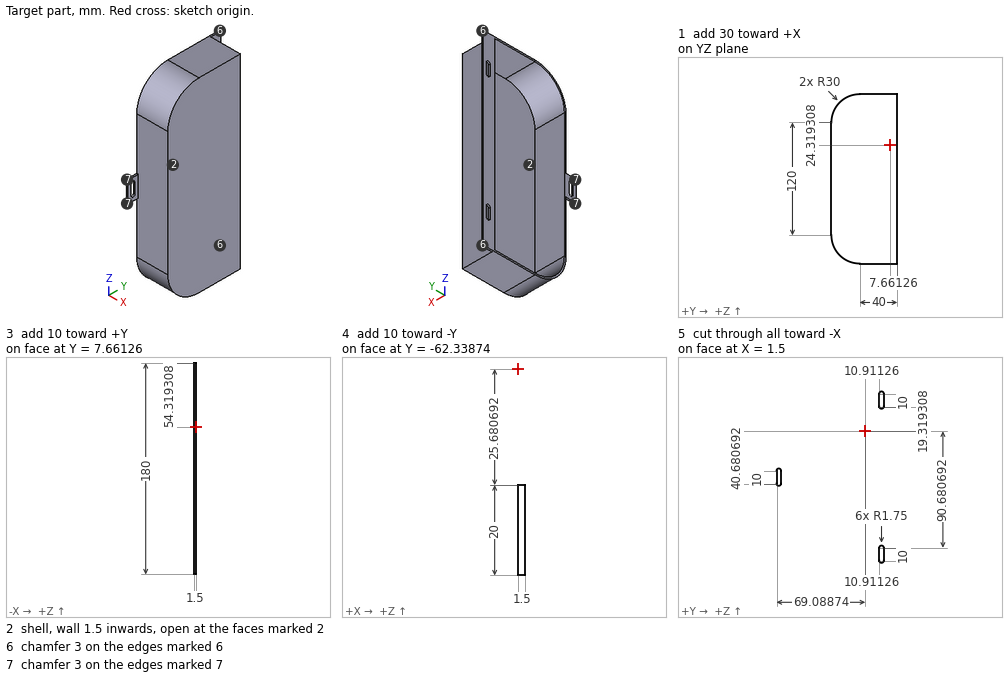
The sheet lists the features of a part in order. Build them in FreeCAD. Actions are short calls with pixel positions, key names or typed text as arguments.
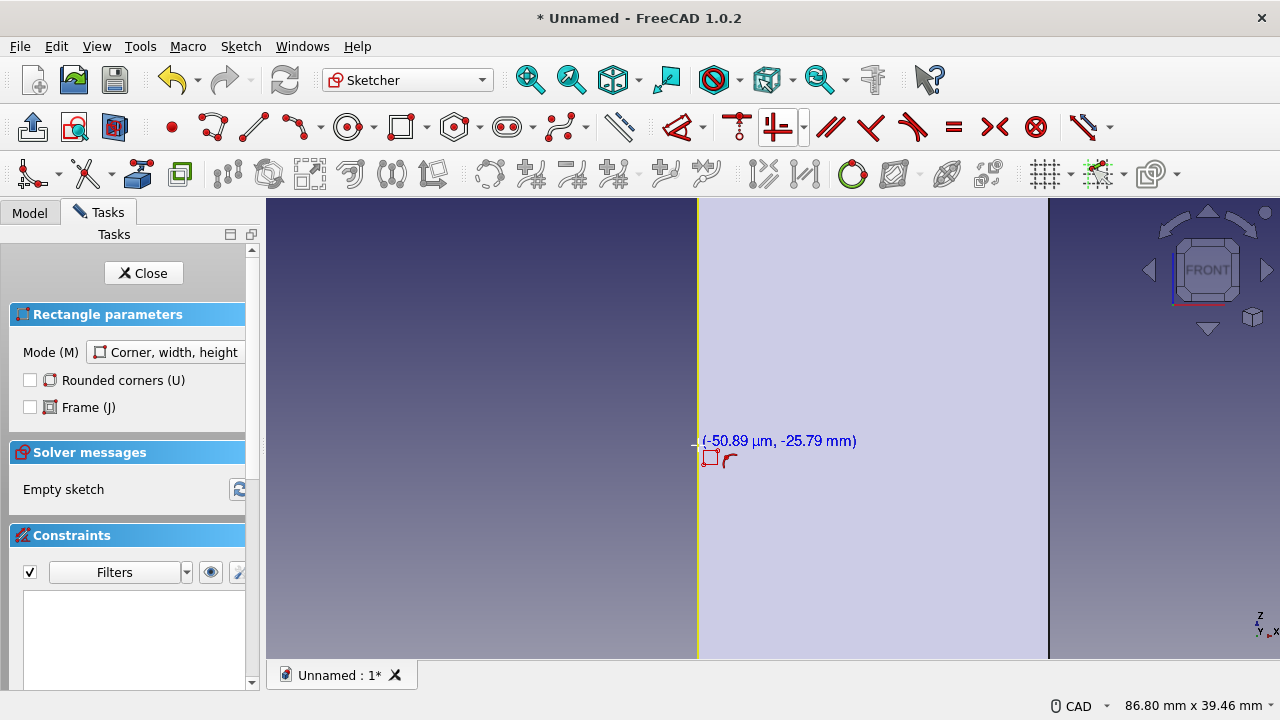
click(698, 445)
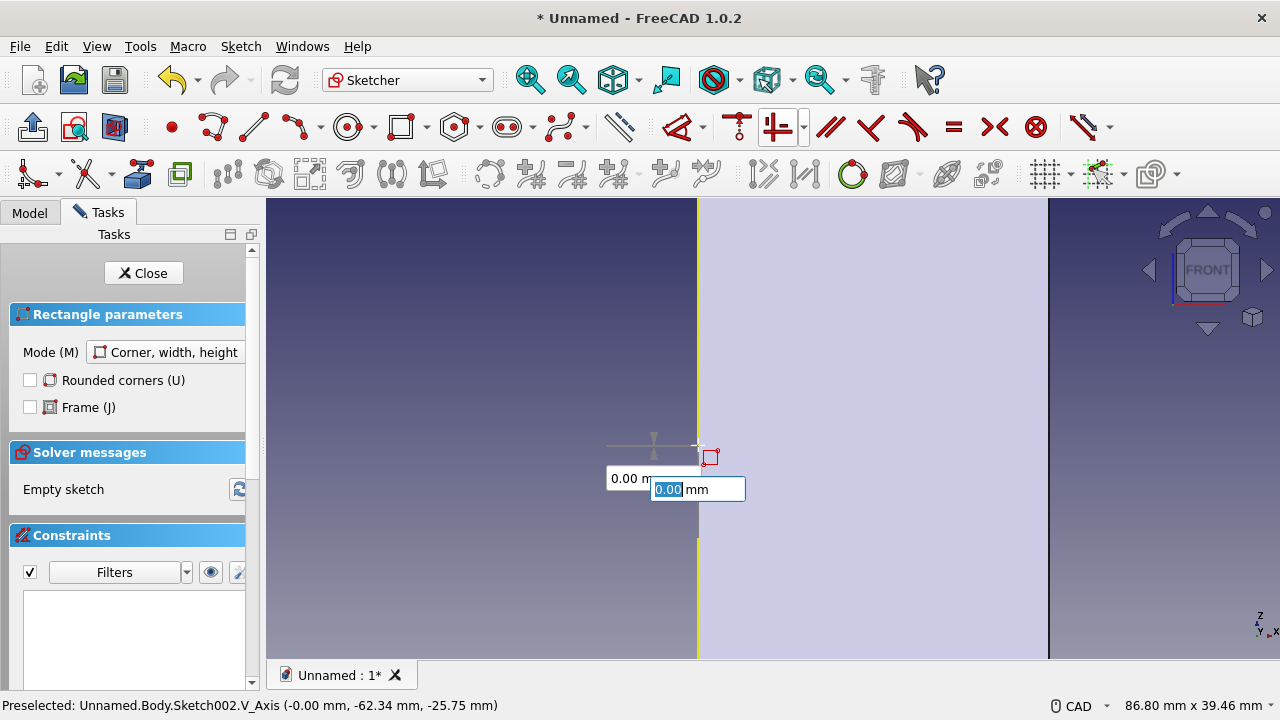
scroll(701, 449, down, 3)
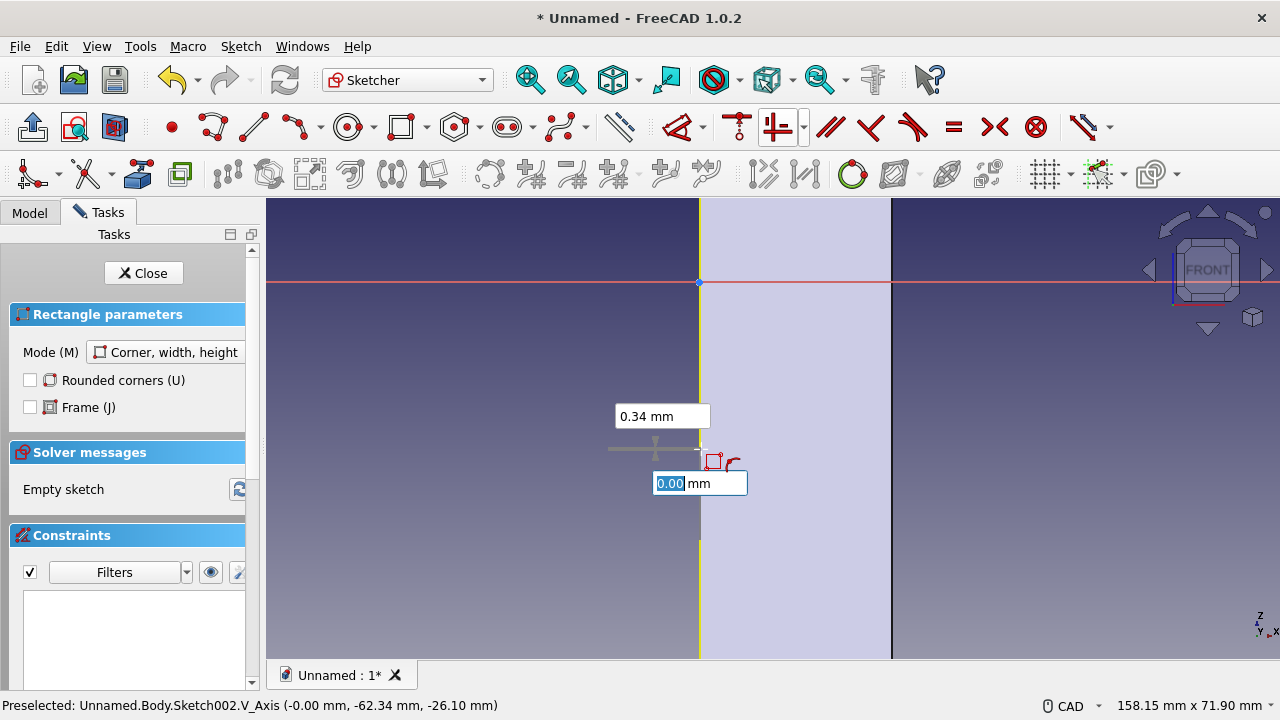
scroll(709, 575, up, 3)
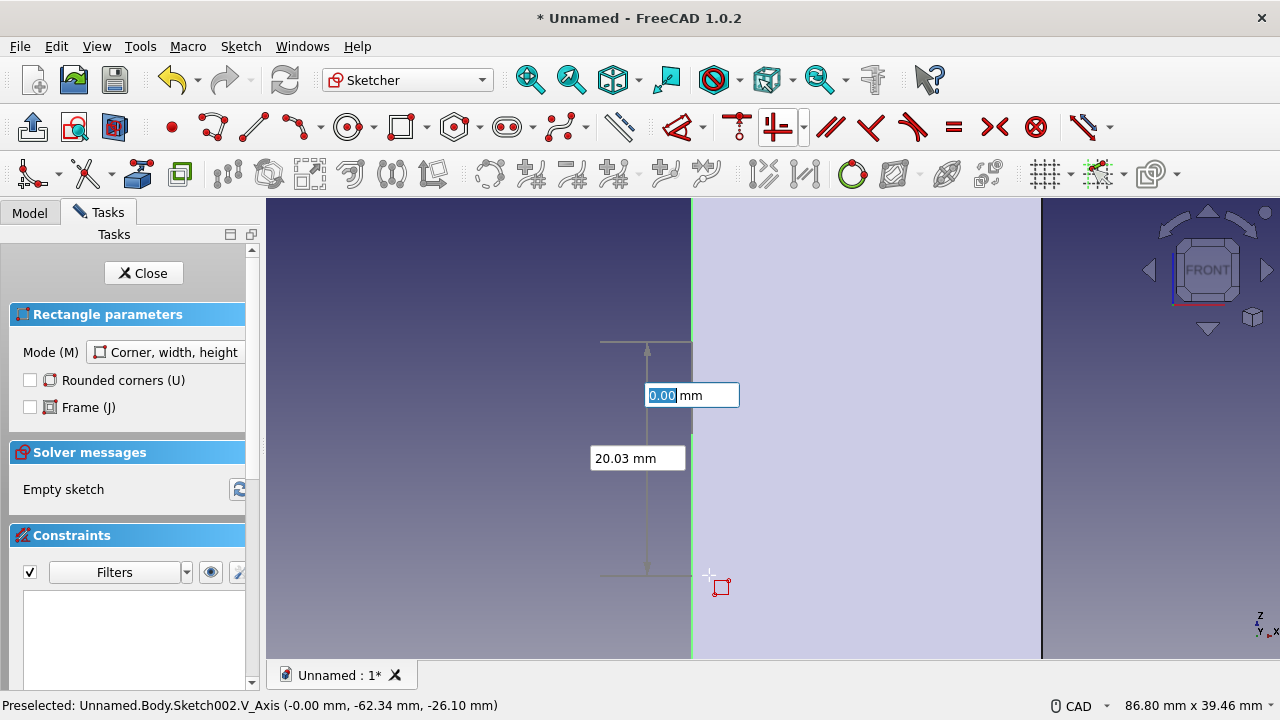
click(709, 575)
key(Escape)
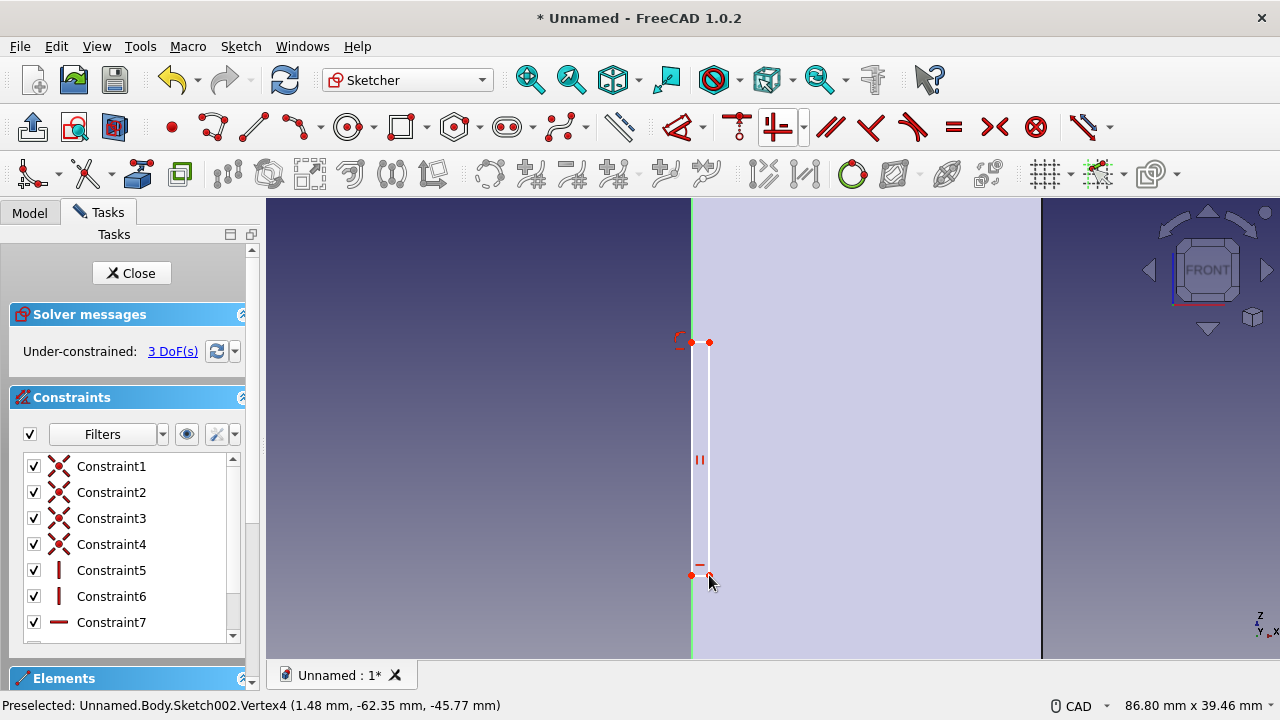
click(676, 128)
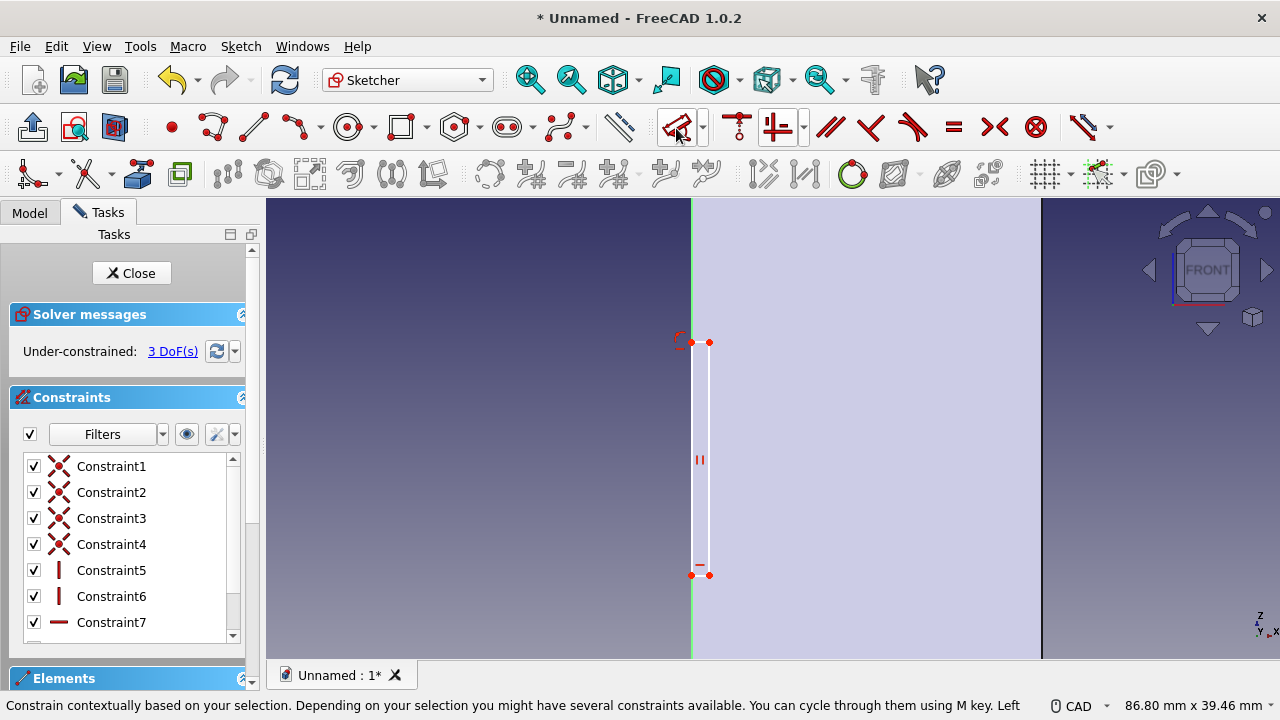
click(692, 412)
click(658, 459)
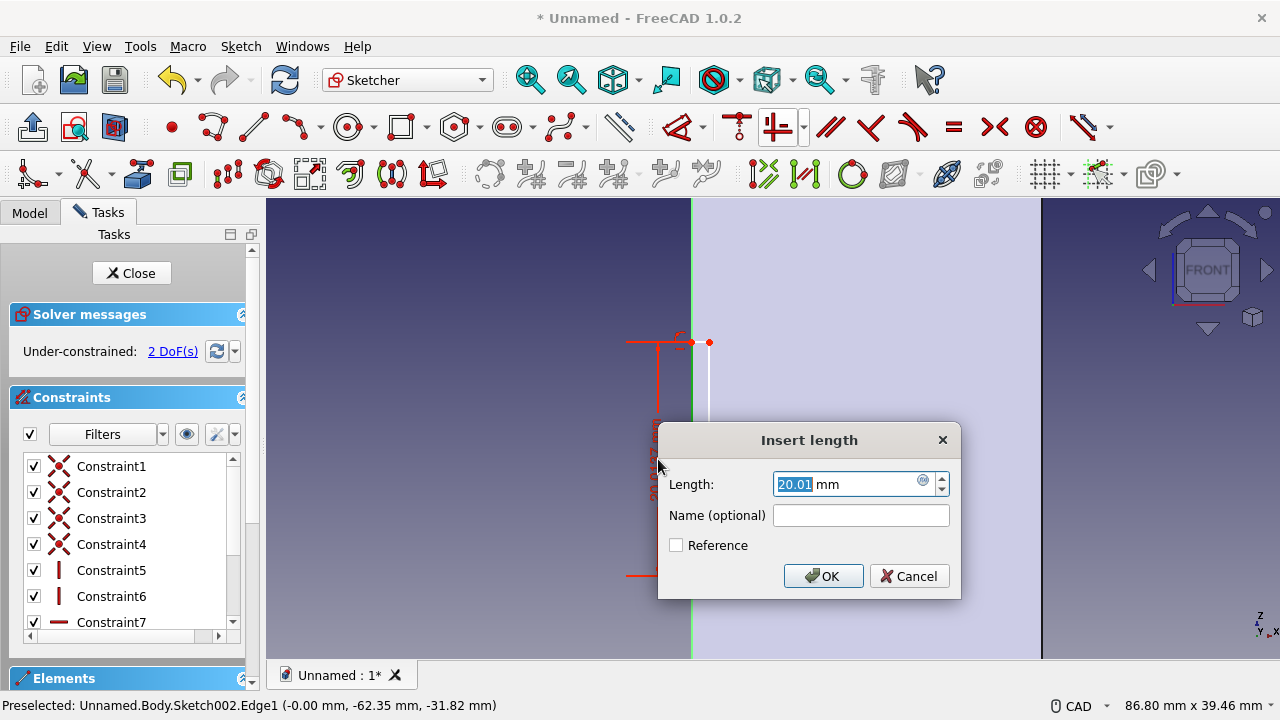
text(20)
key(Return)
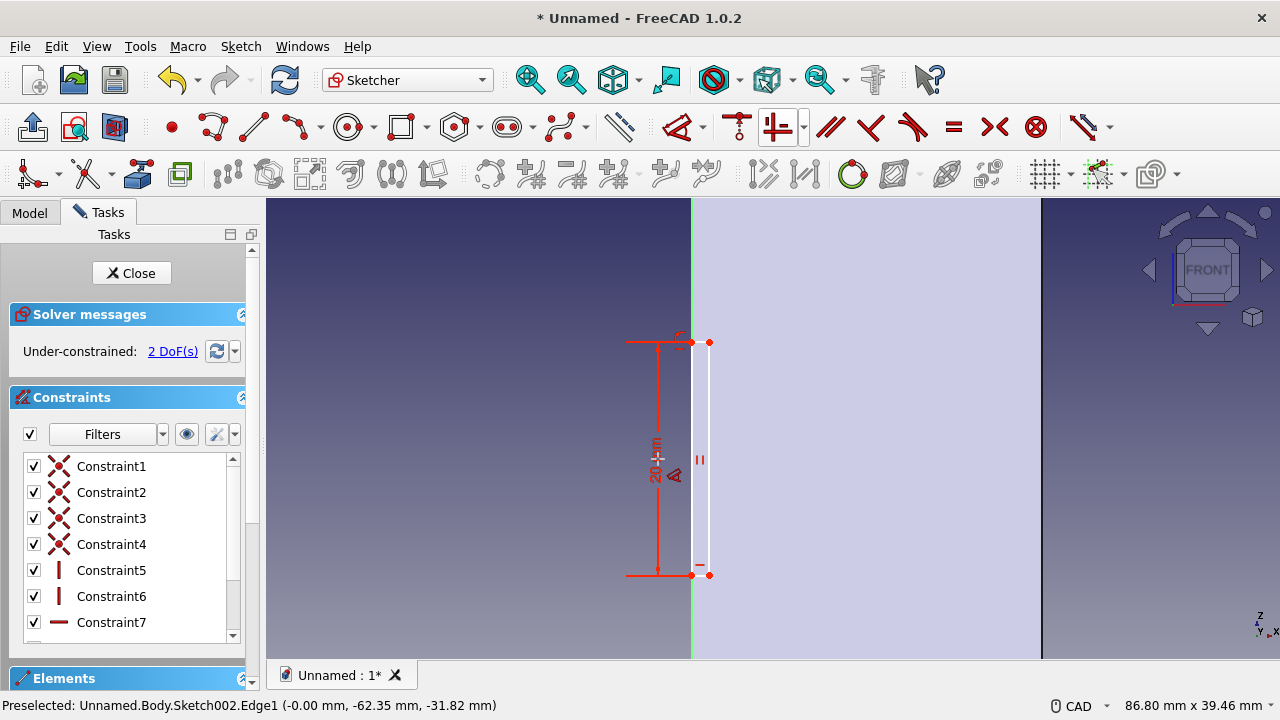
scroll(700, 576, up, 5)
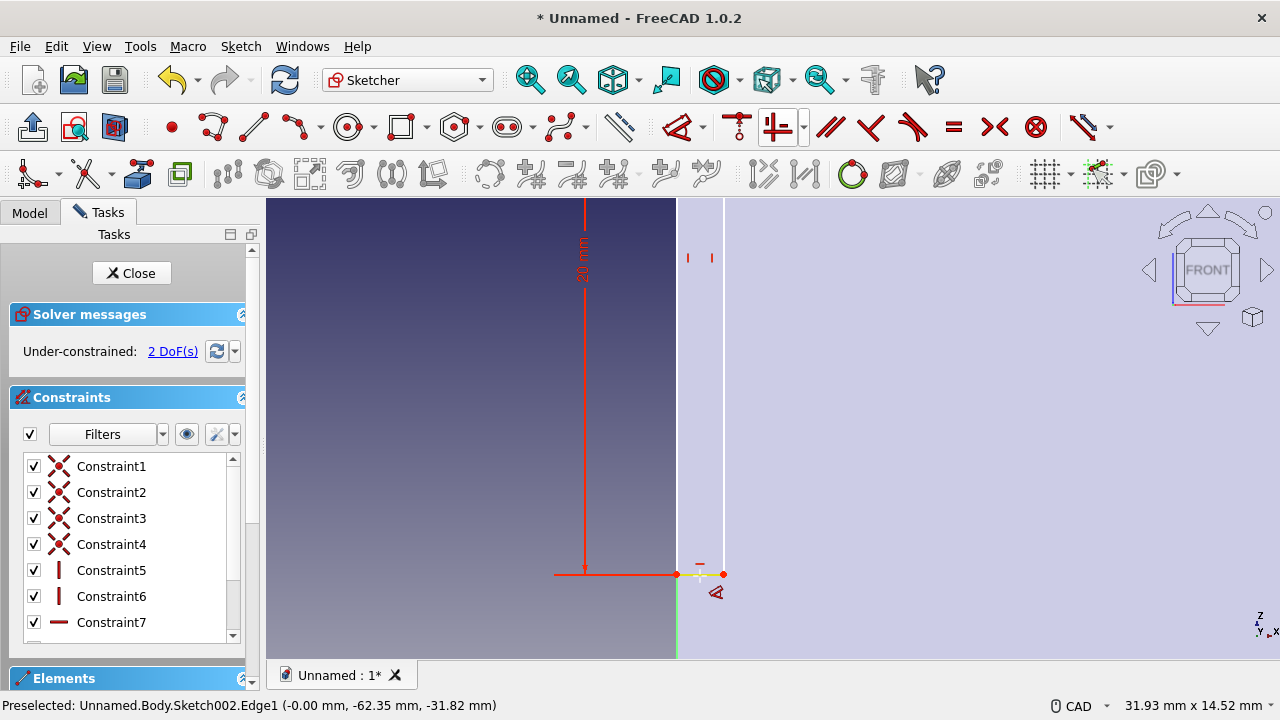
click(700, 575)
click(700, 609)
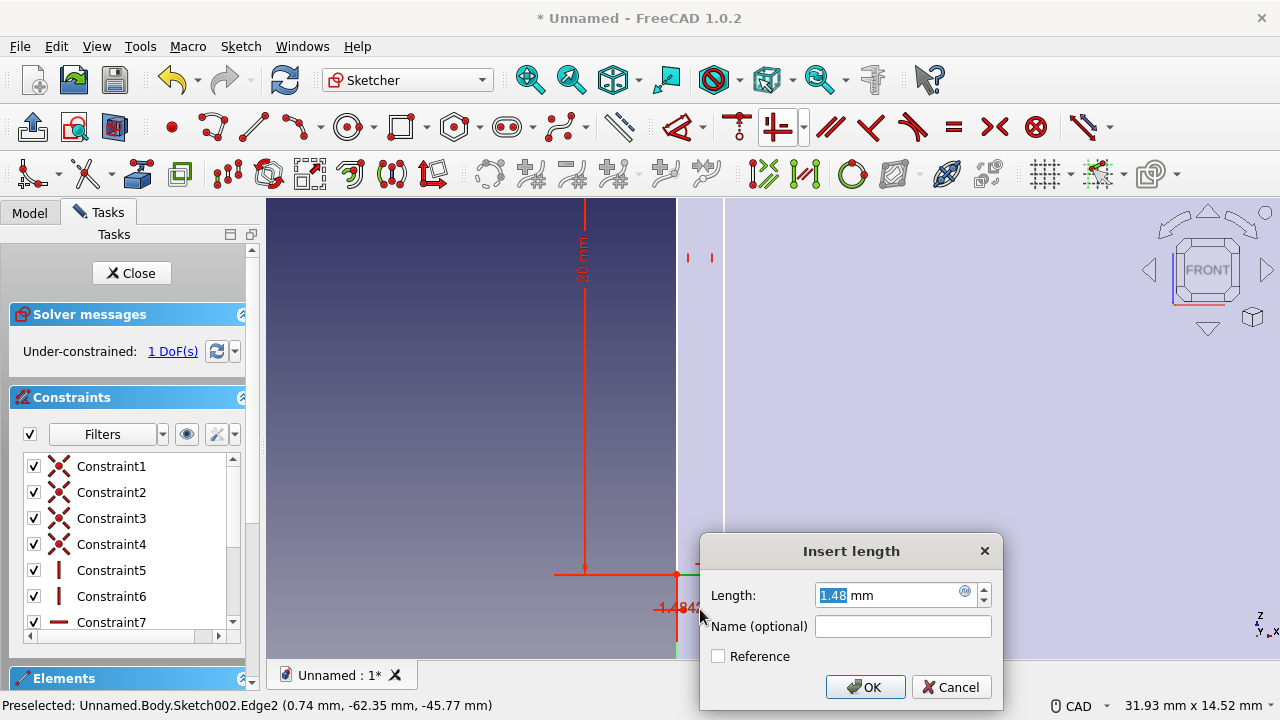
text(1.5)
key(Return)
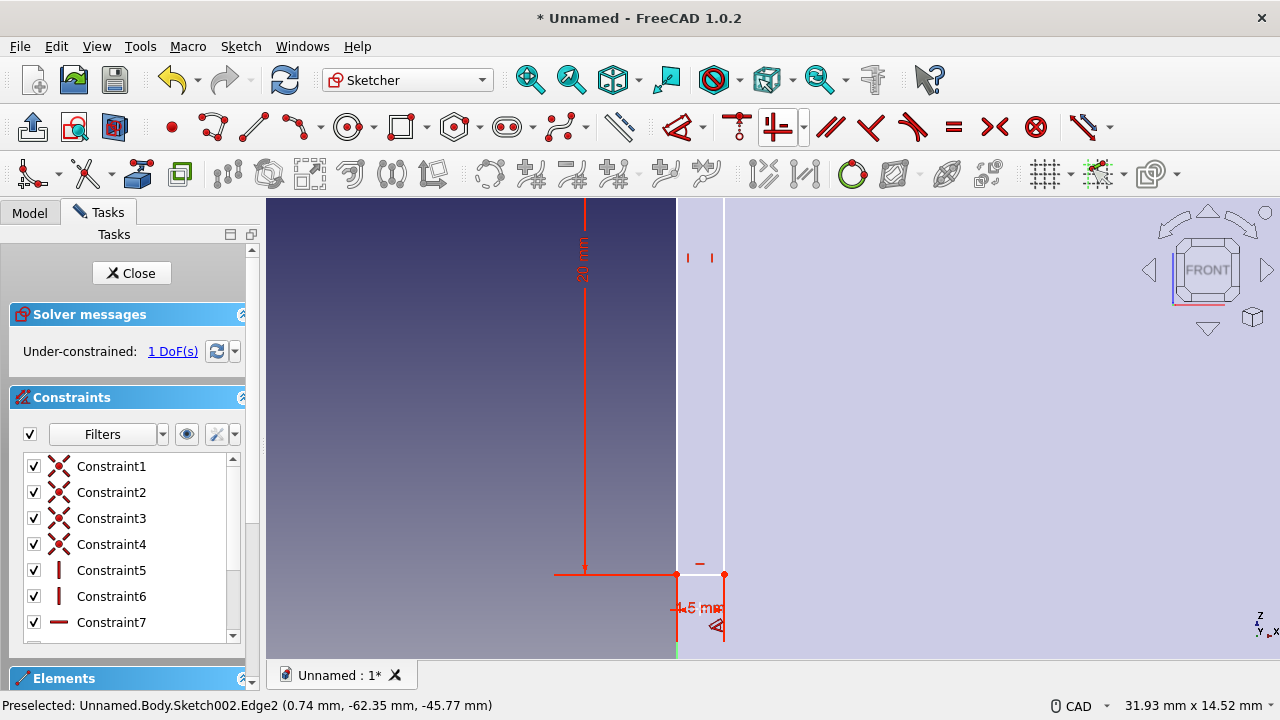
scroll(706, 576, down, 8)